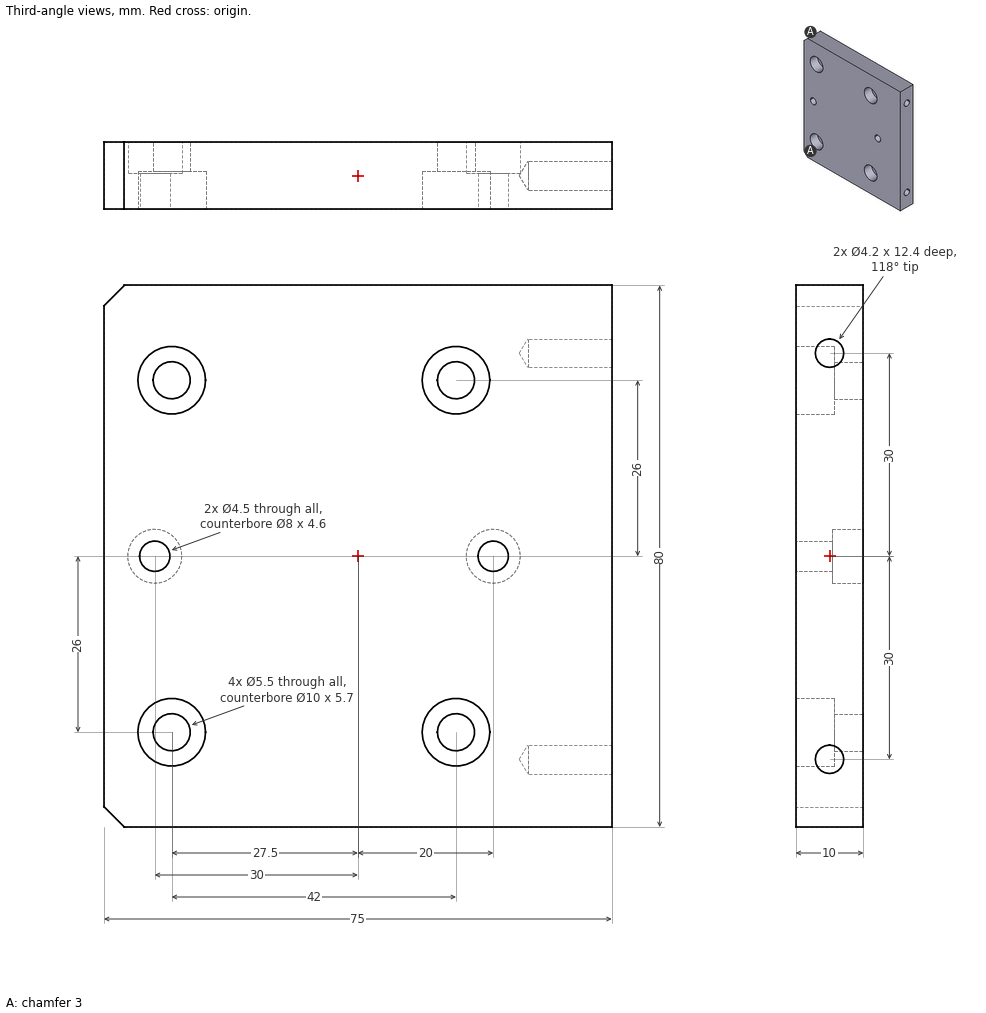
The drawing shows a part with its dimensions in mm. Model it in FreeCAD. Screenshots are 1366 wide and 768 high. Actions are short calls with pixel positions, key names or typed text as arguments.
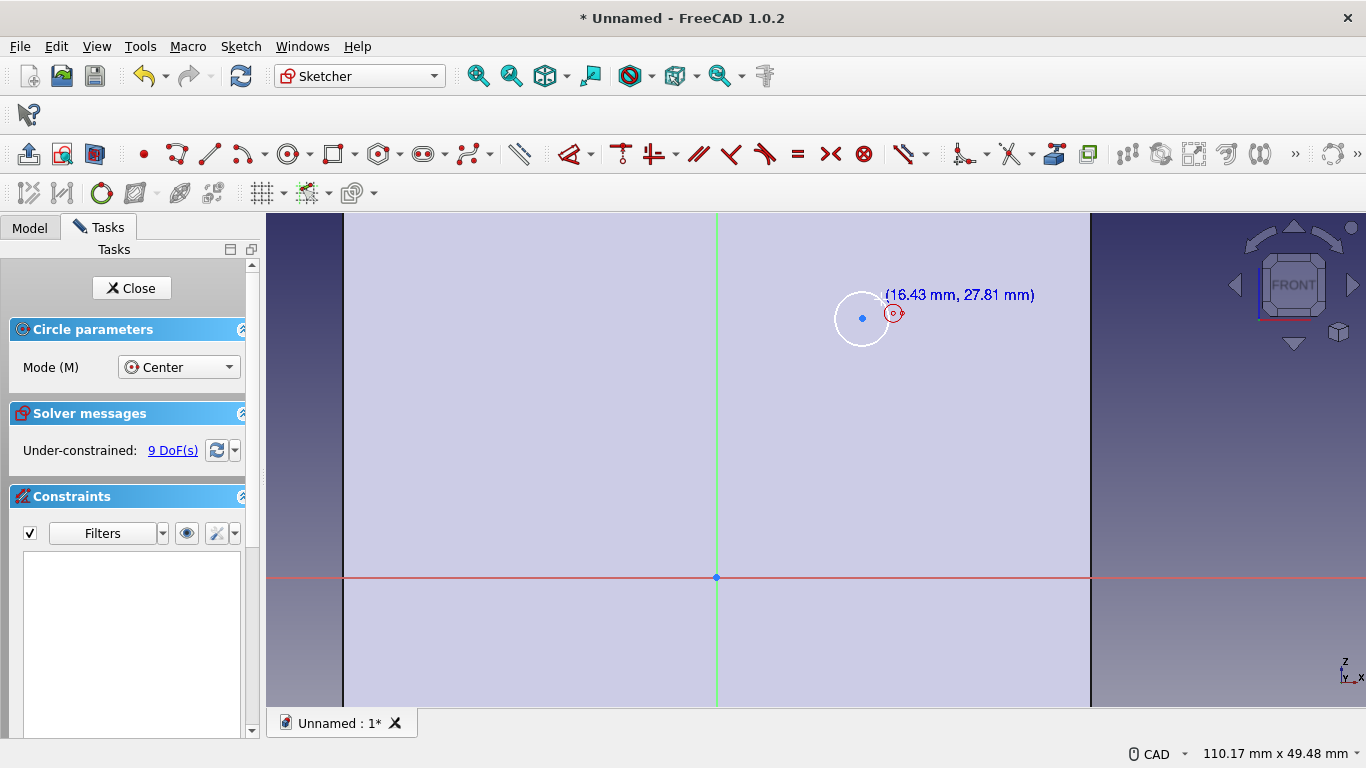
click(442, 318)
click(462, 299)
key(Escape)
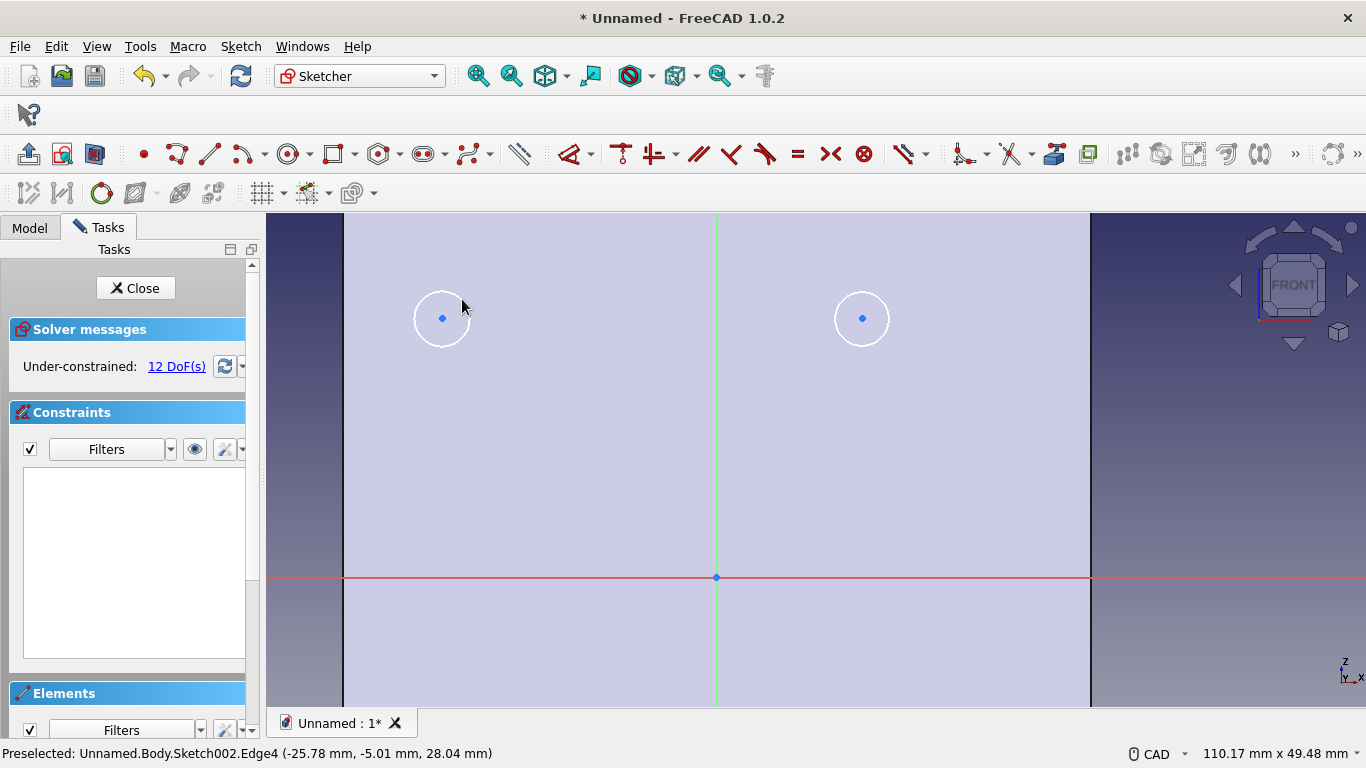
scroll(864, 317, down, 3)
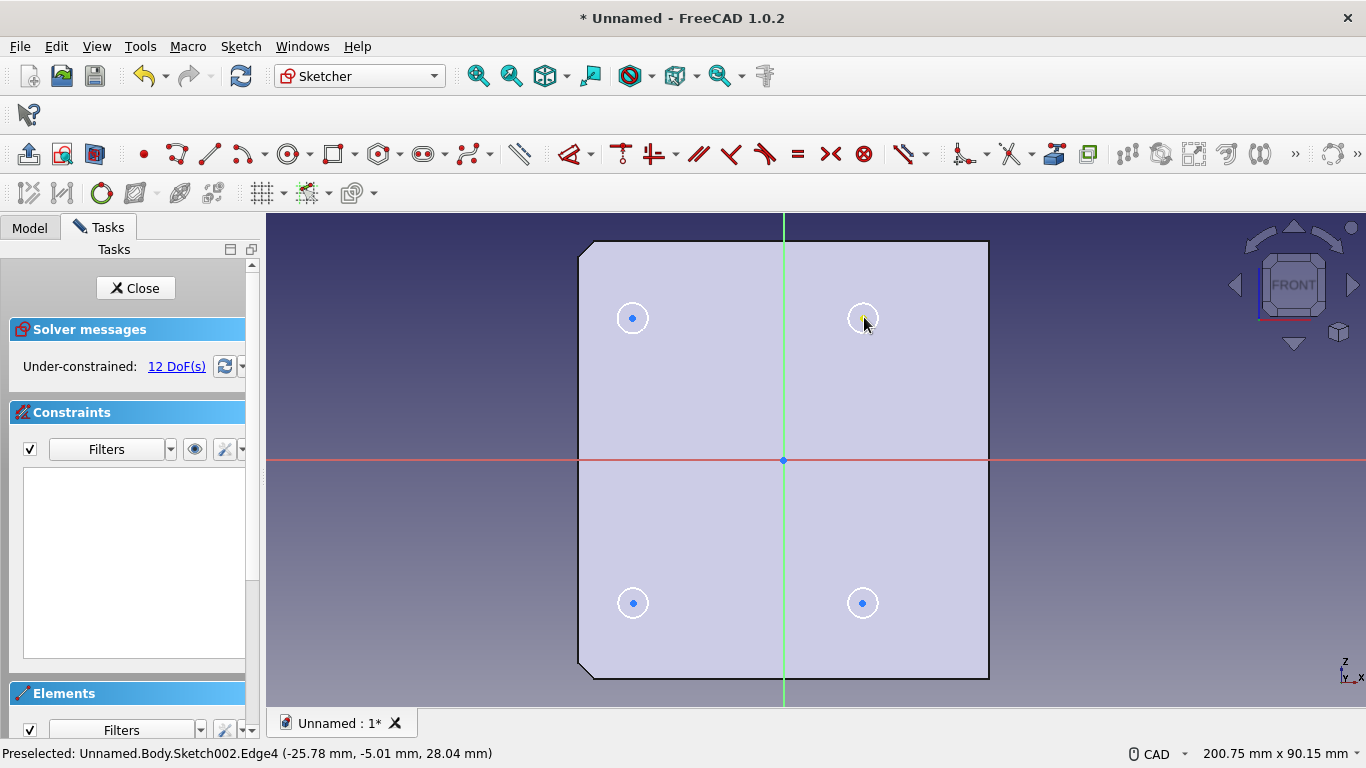
click(643, 593)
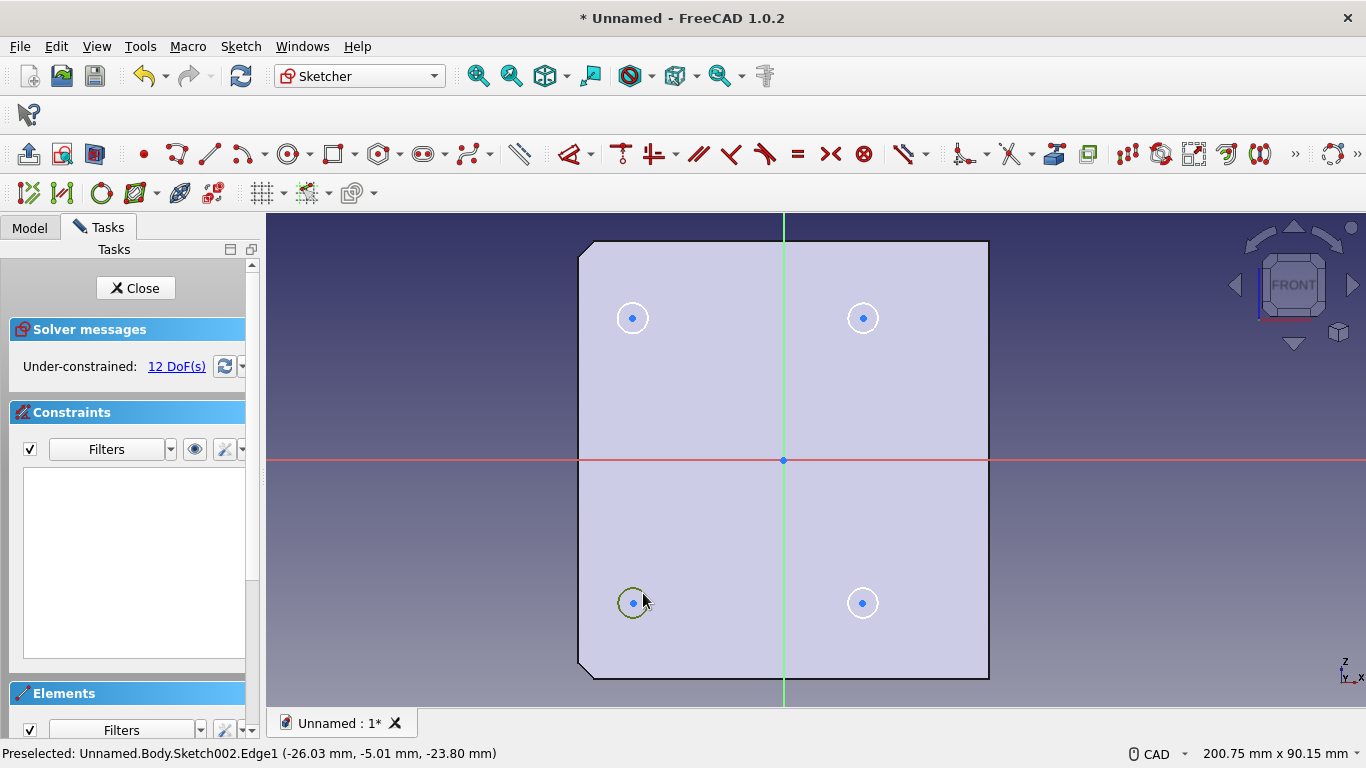
click(873, 593)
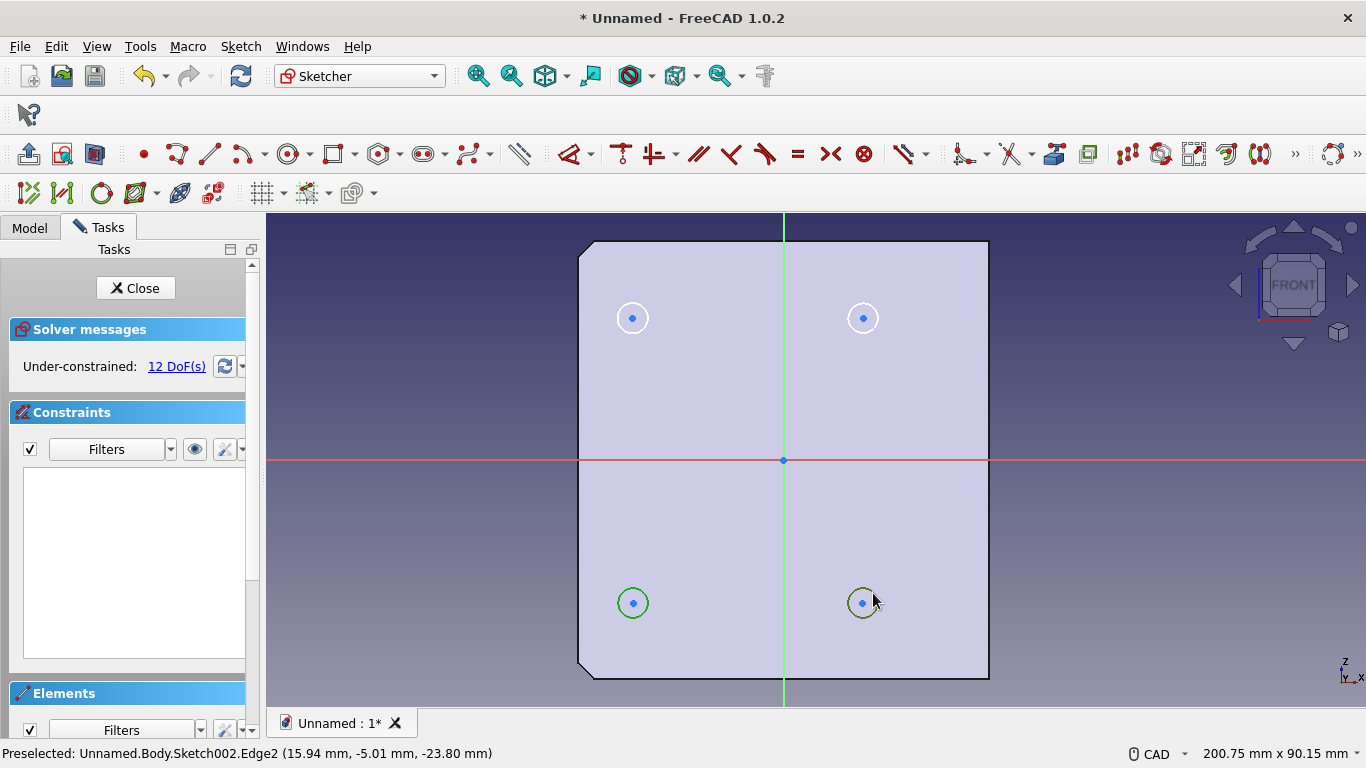
click(874, 308)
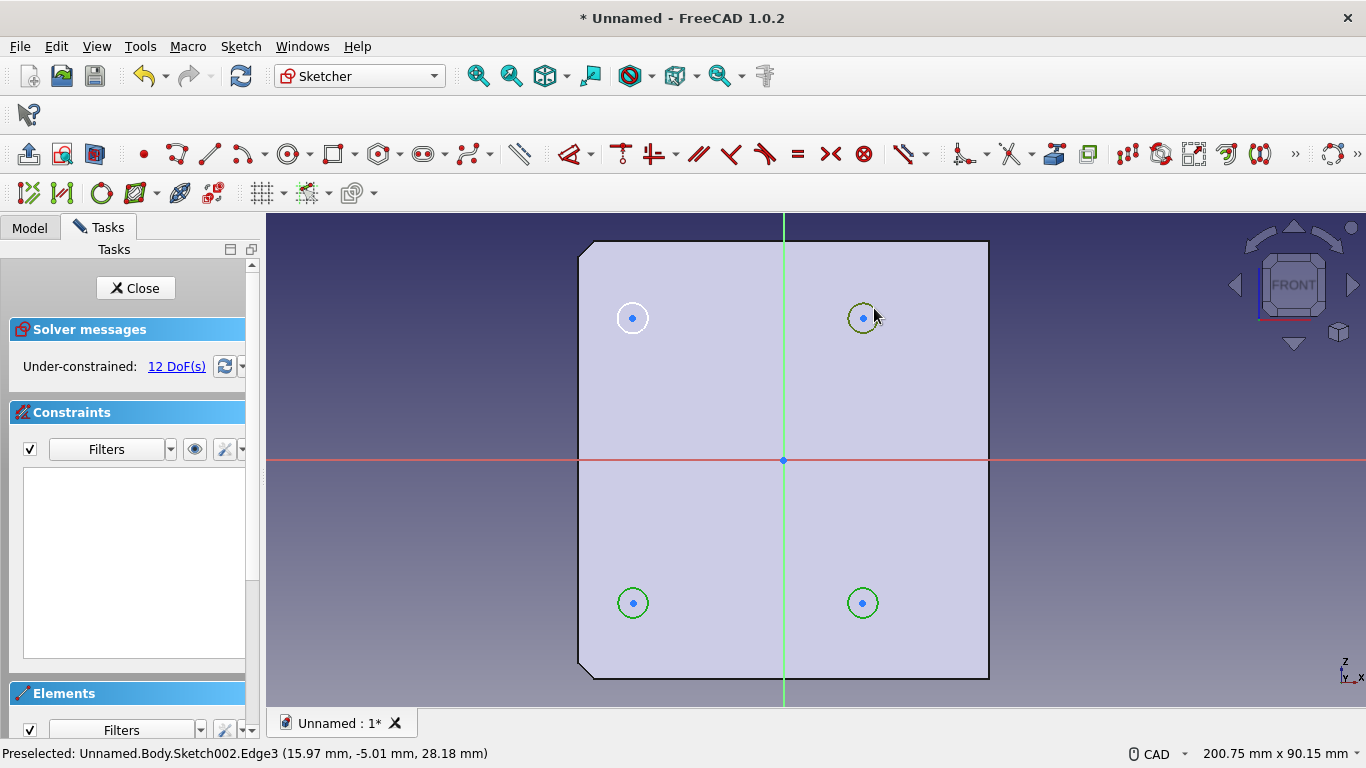
click(643, 307)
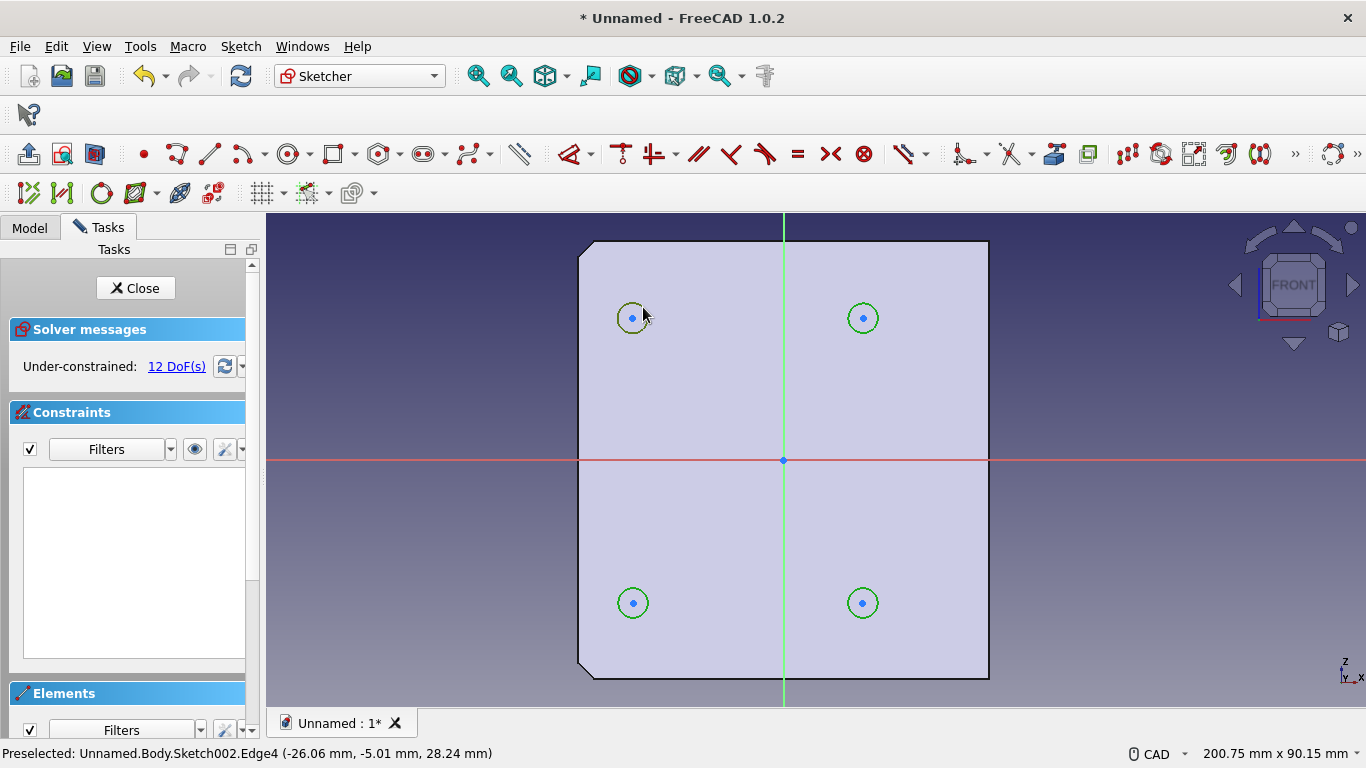
click(798, 154)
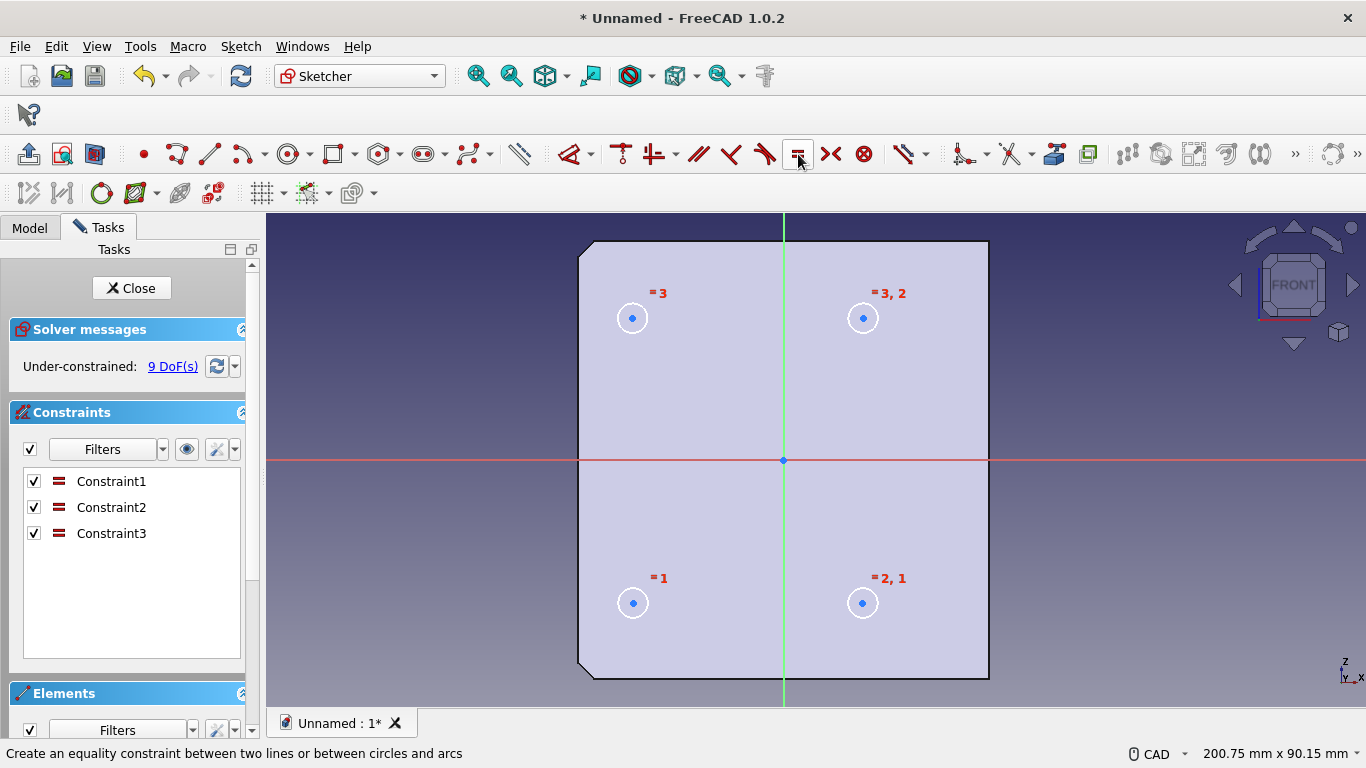
click(633, 603)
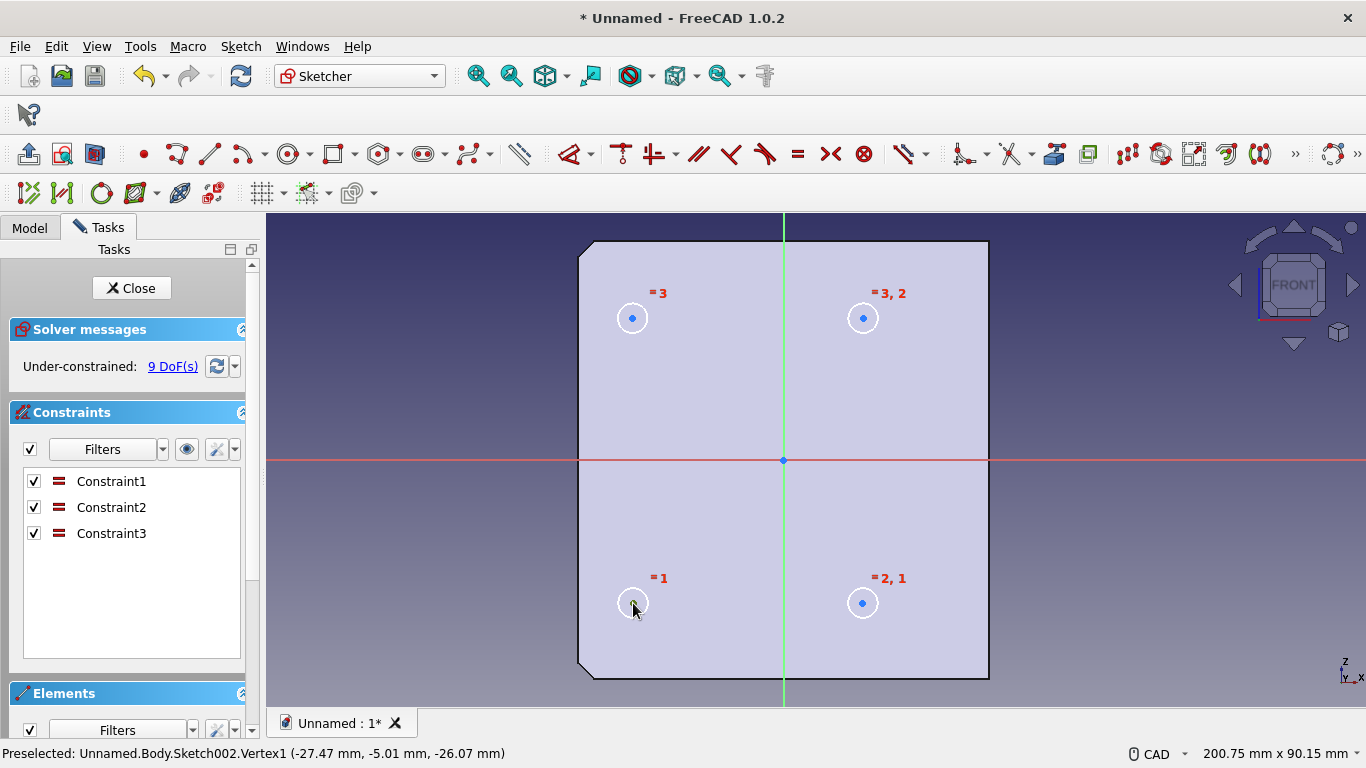
click(863, 603)